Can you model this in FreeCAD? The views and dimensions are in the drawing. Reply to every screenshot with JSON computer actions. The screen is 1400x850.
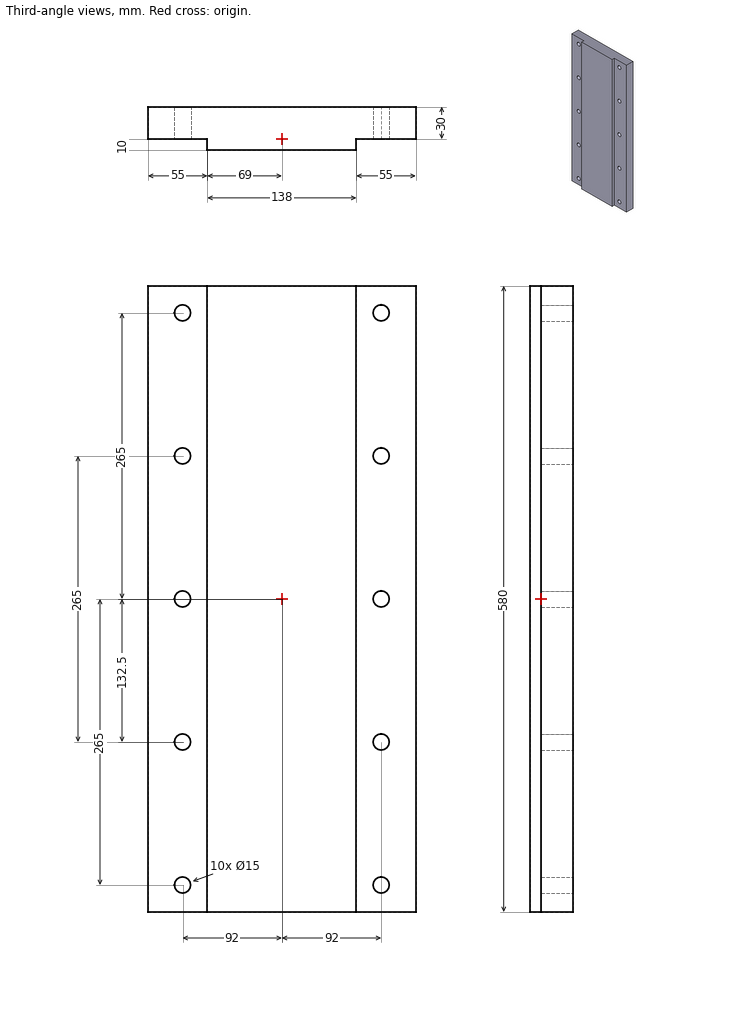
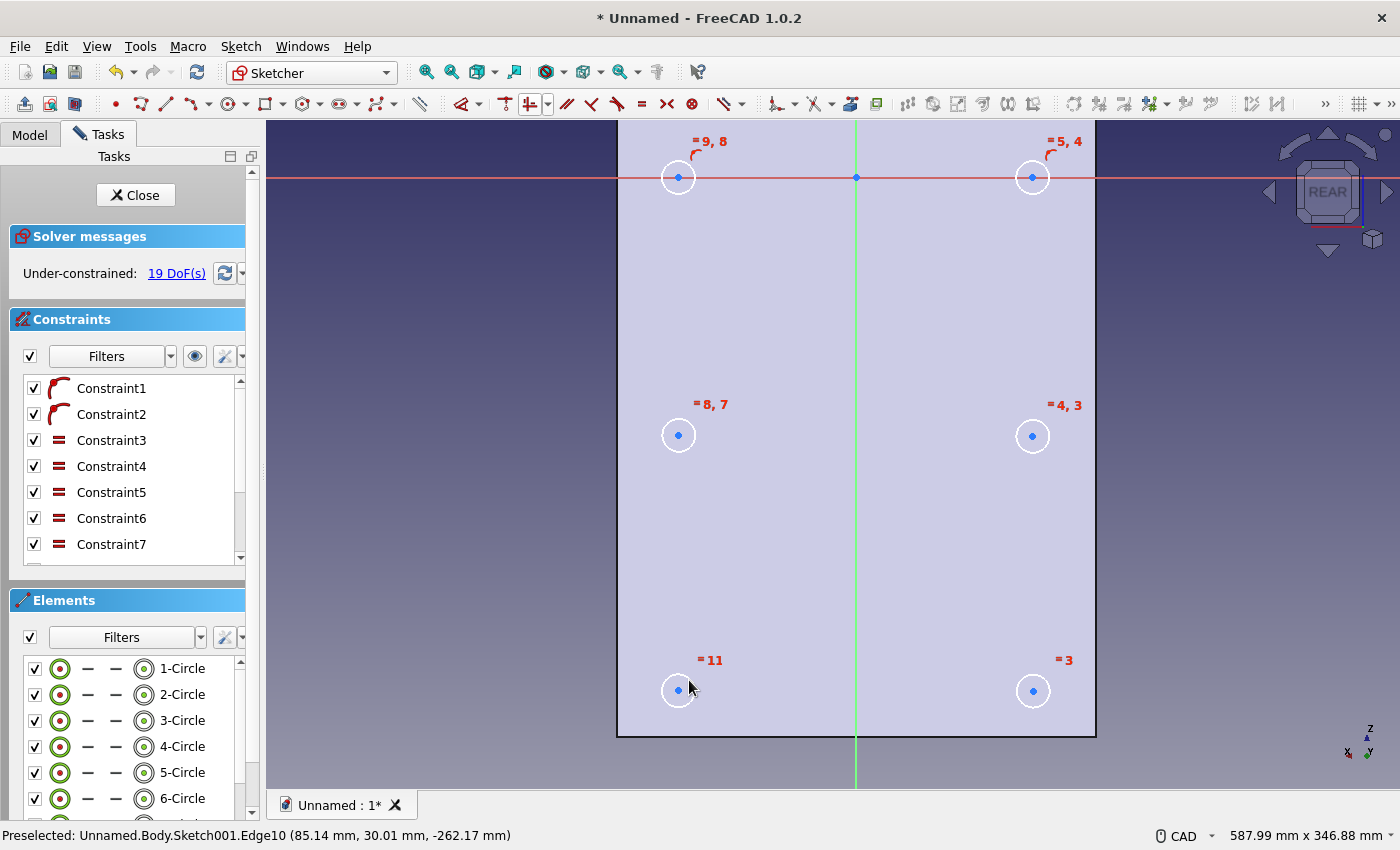
{"action": "left_click", "coordinate": [1033, 691]}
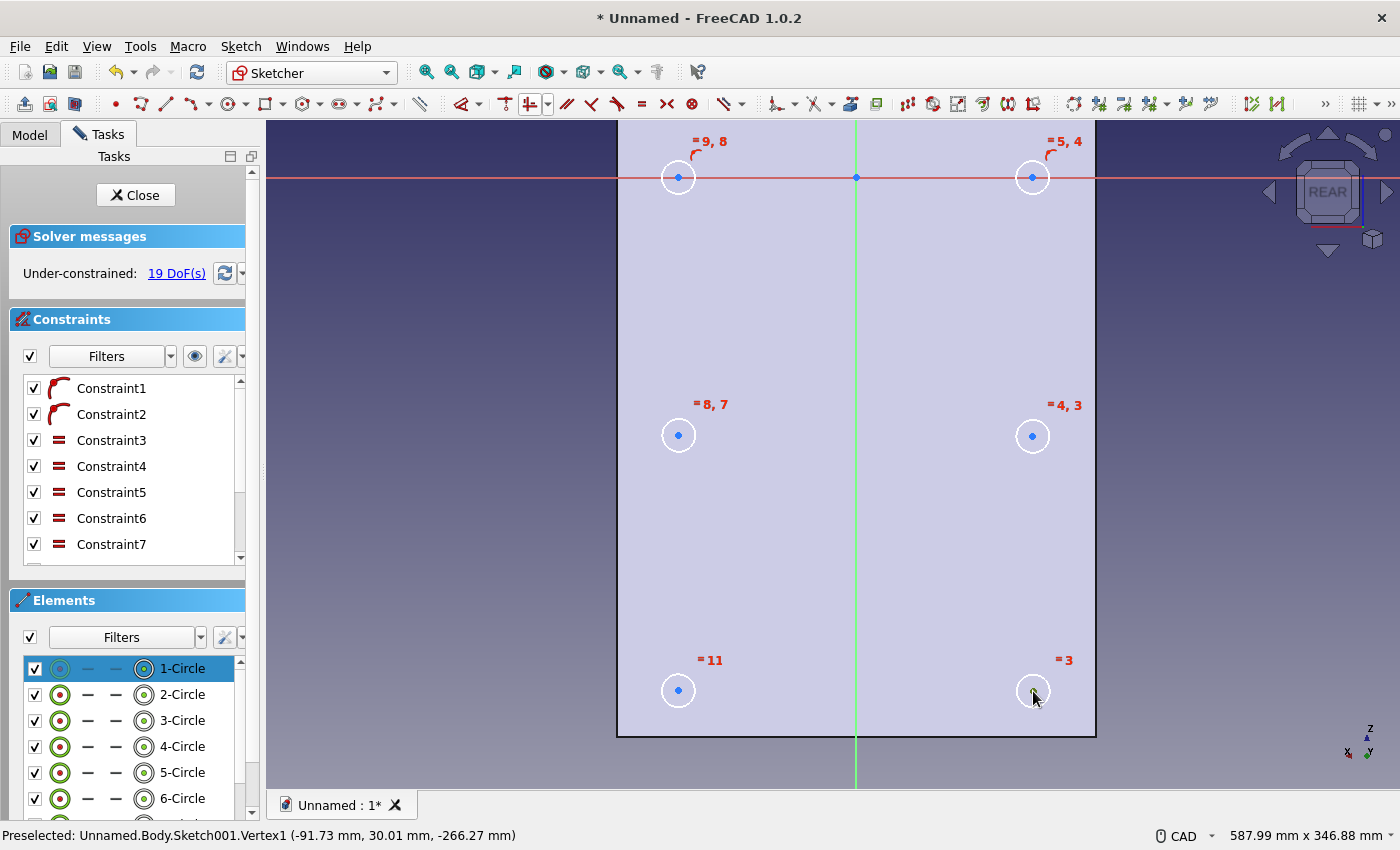
{"action": "left_click", "coordinate": [1033, 436]}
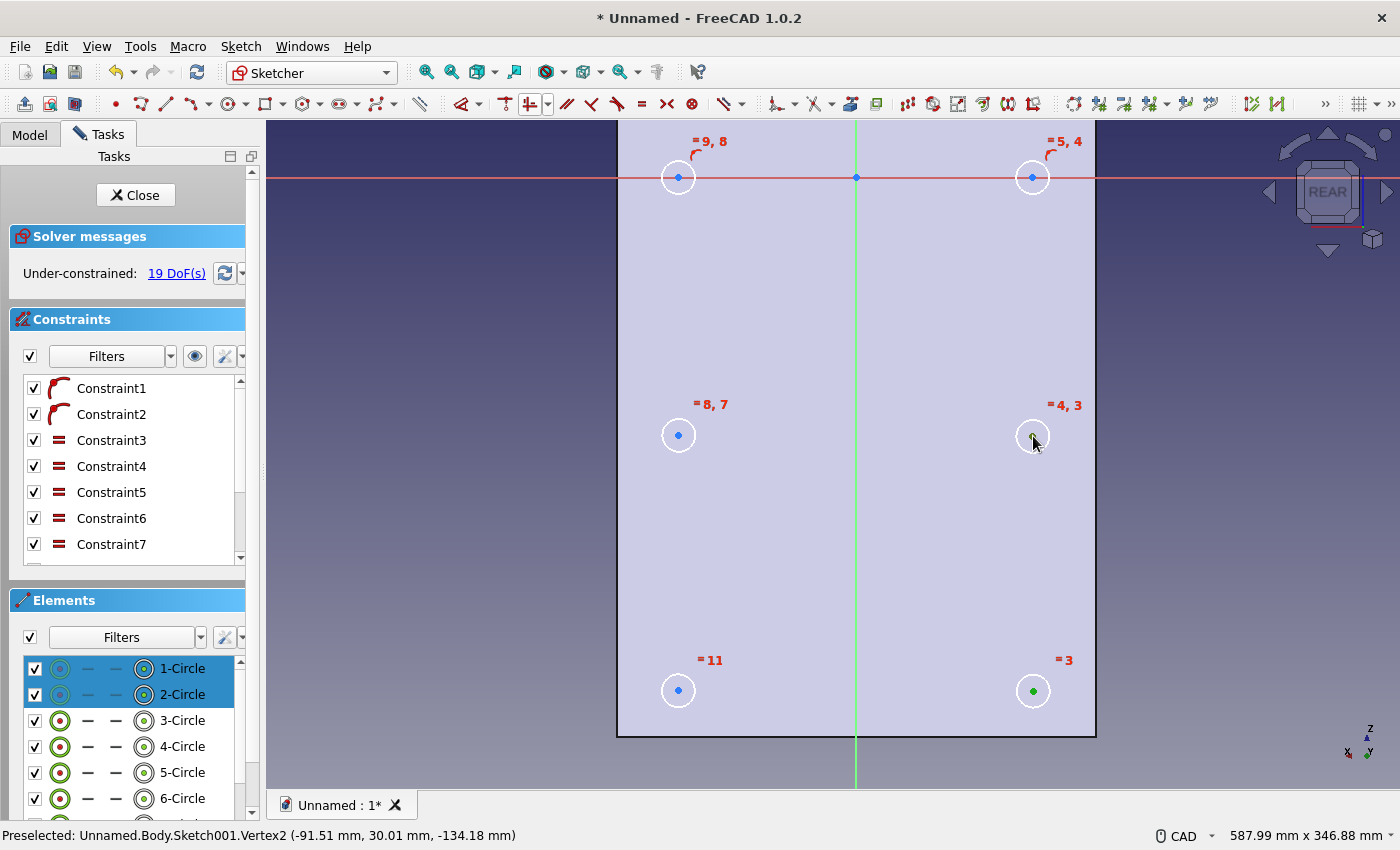
{"action": "left_click", "coordinate": [548, 104]}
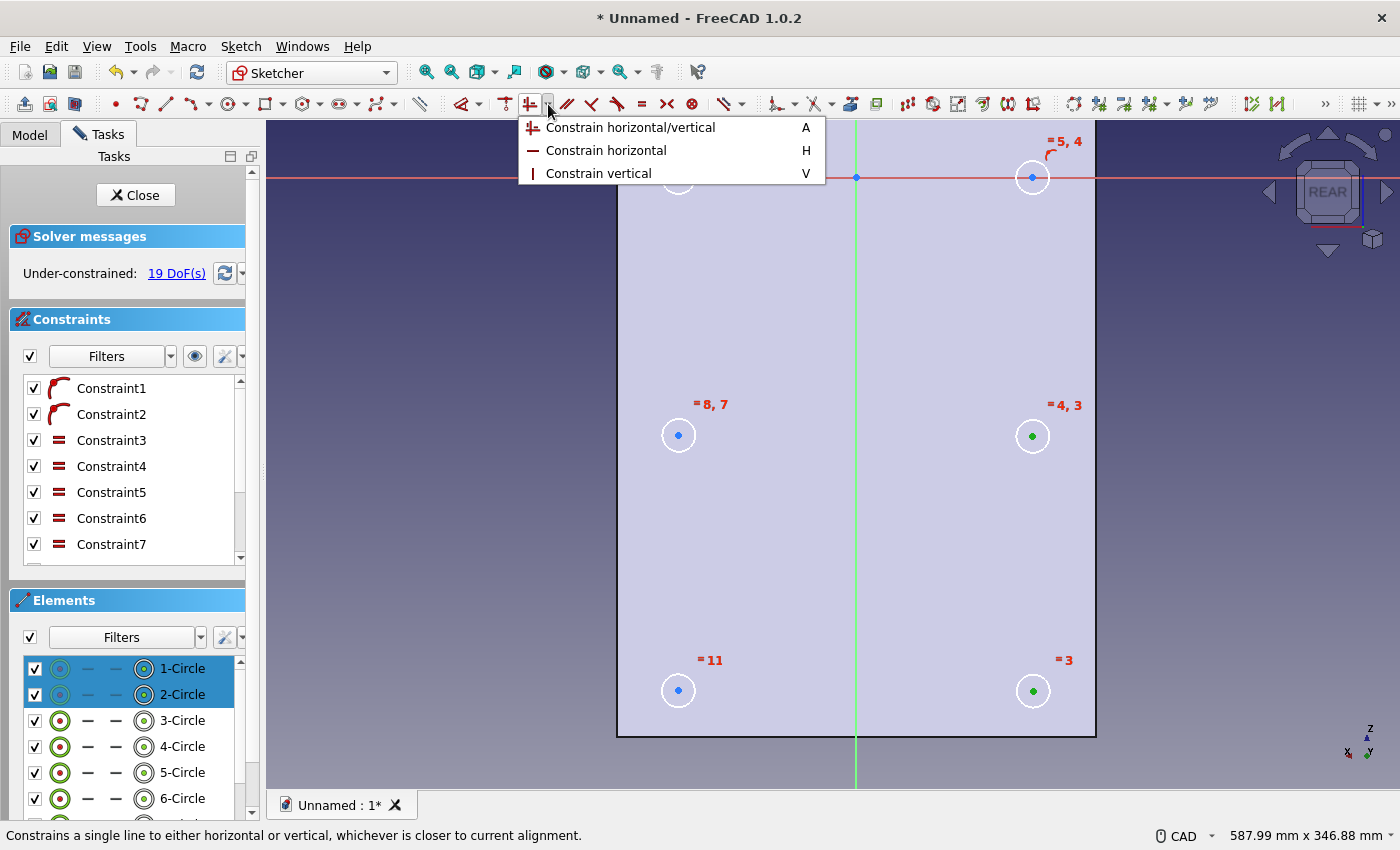
{"action": "left_click", "coordinate": [672, 174]}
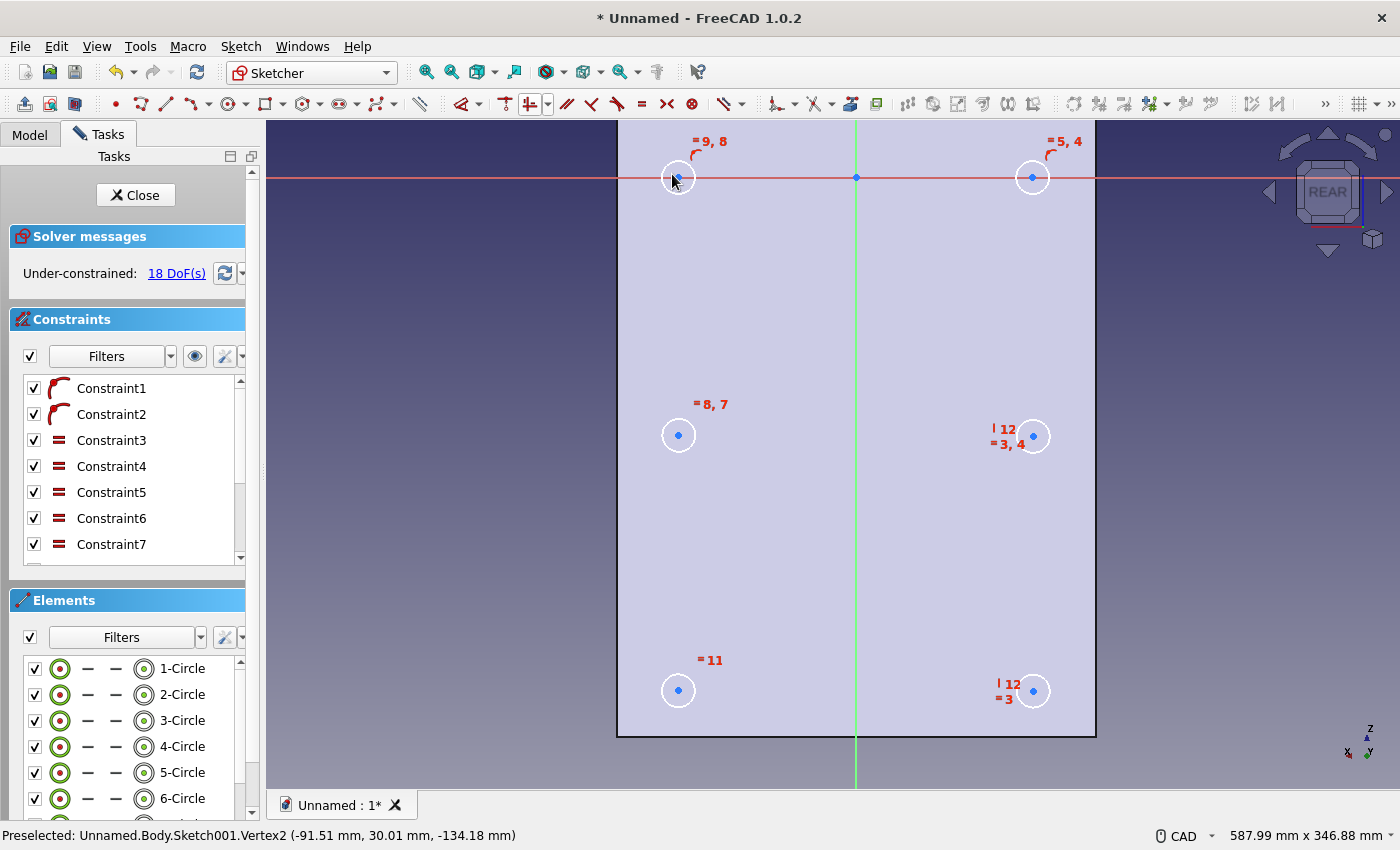
{"action": "left_click", "coordinate": [1033, 436]}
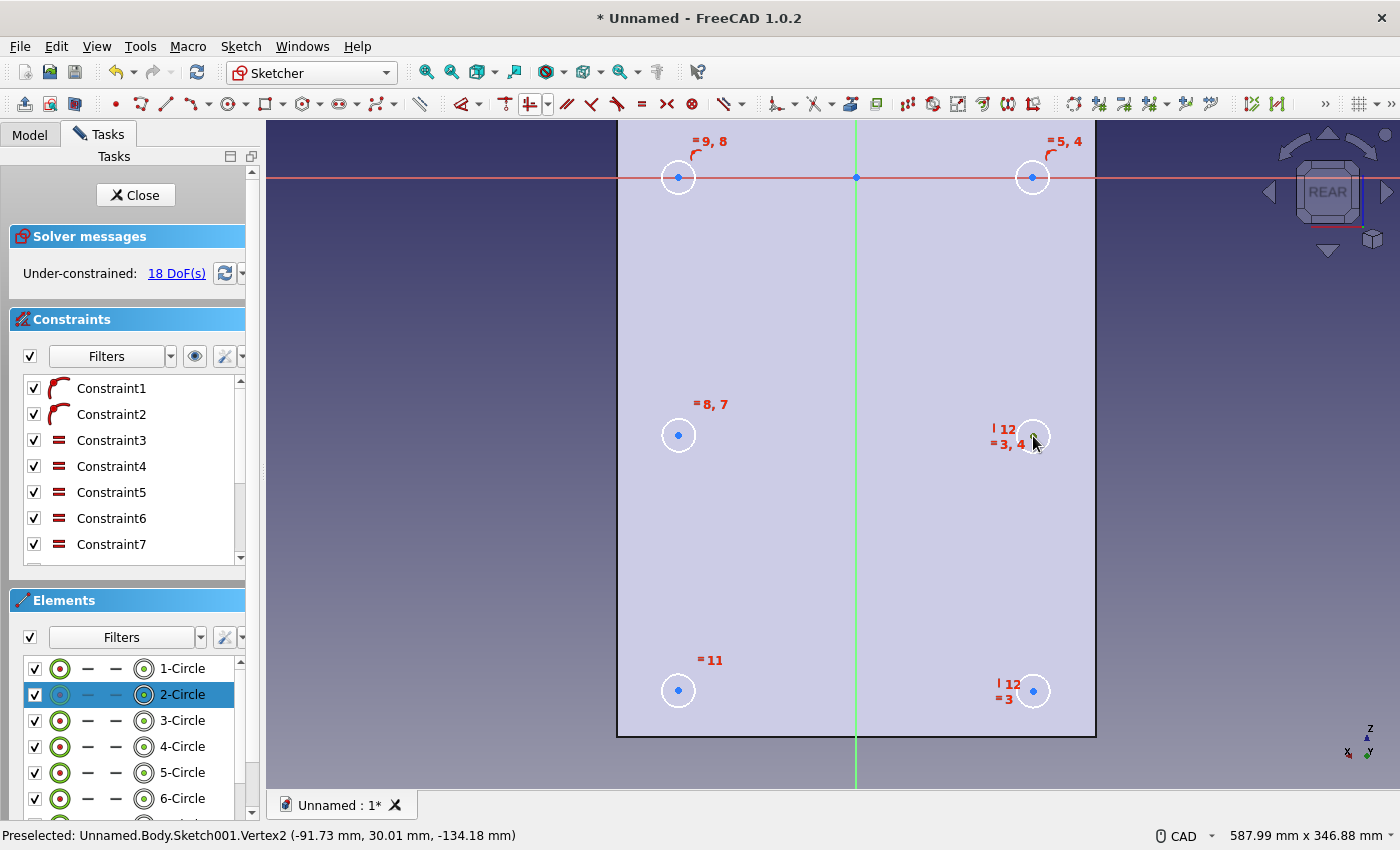
{"action": "left_click", "coordinate": [1033, 178]}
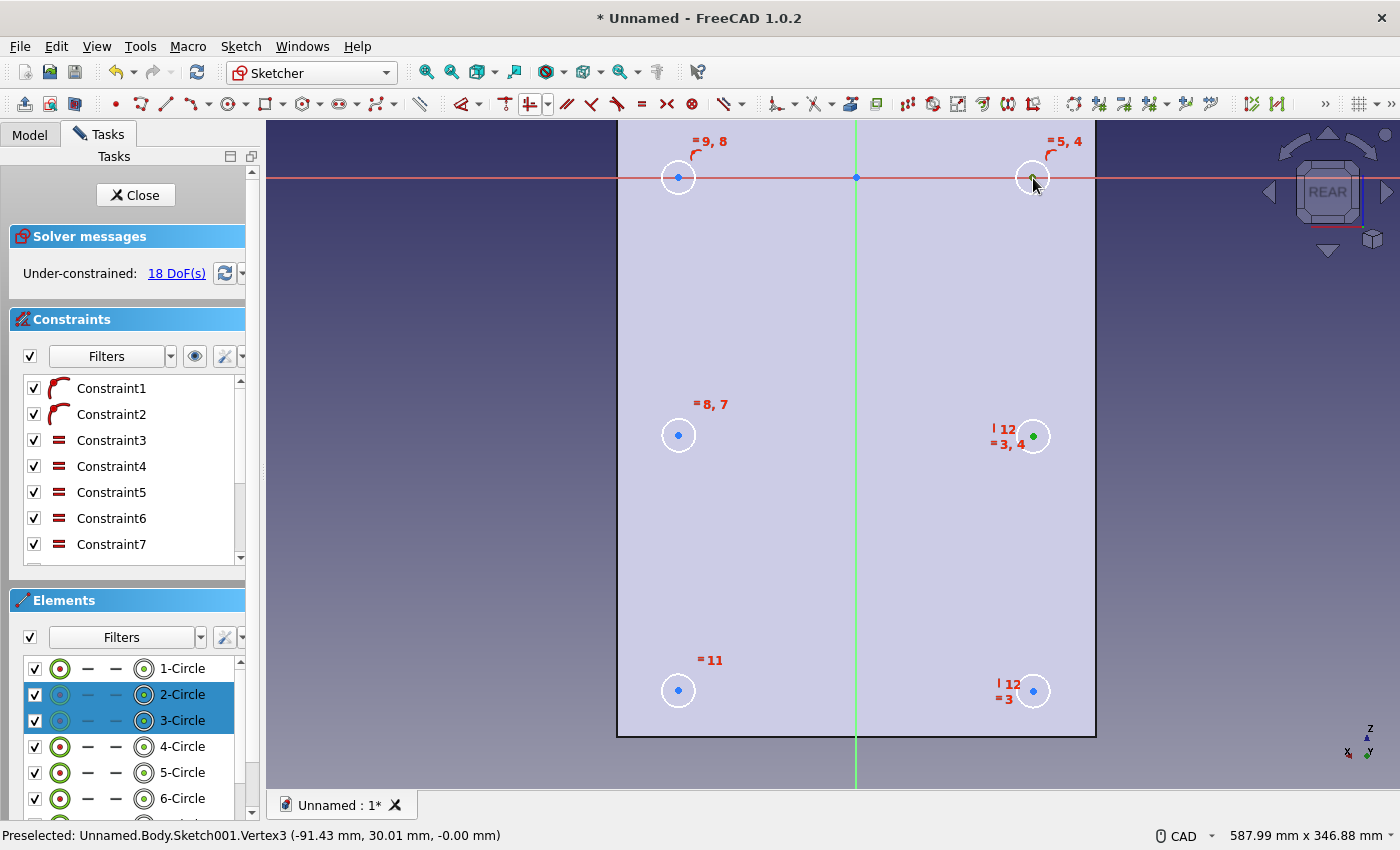
{"action": "key", "text": "v"}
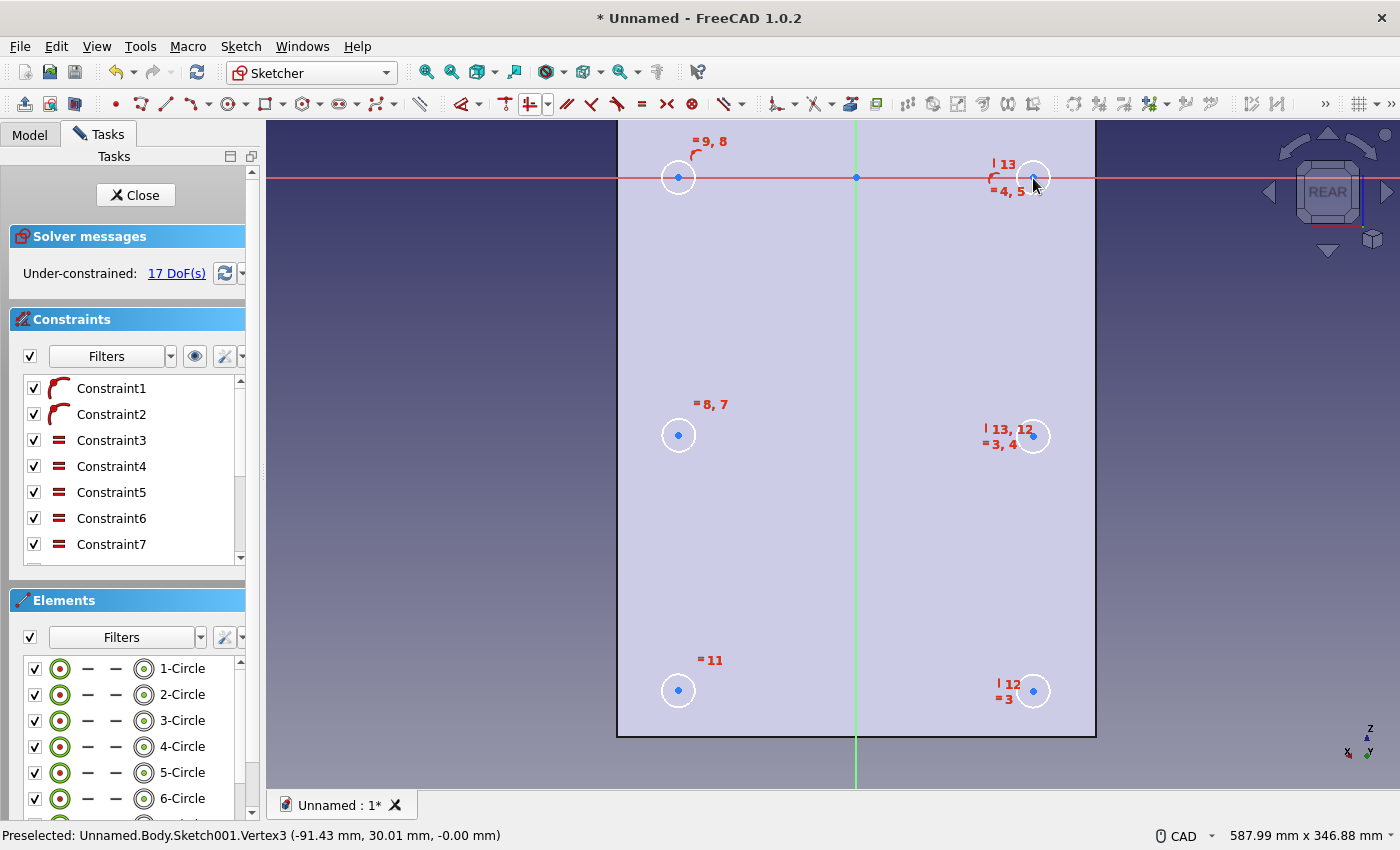
{"action": "left_click", "coordinate": [1033, 178]}